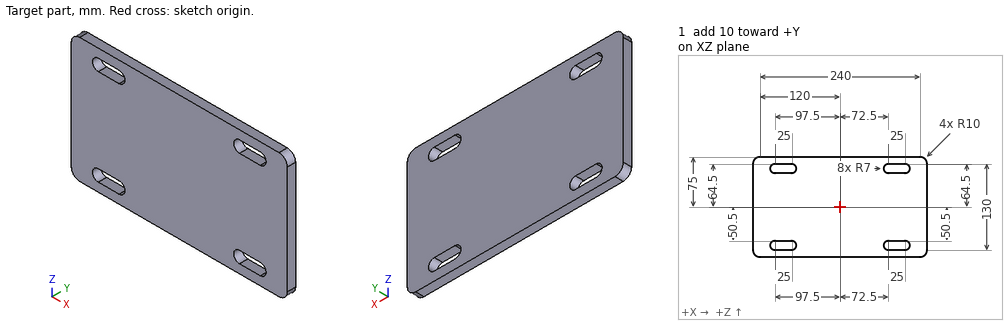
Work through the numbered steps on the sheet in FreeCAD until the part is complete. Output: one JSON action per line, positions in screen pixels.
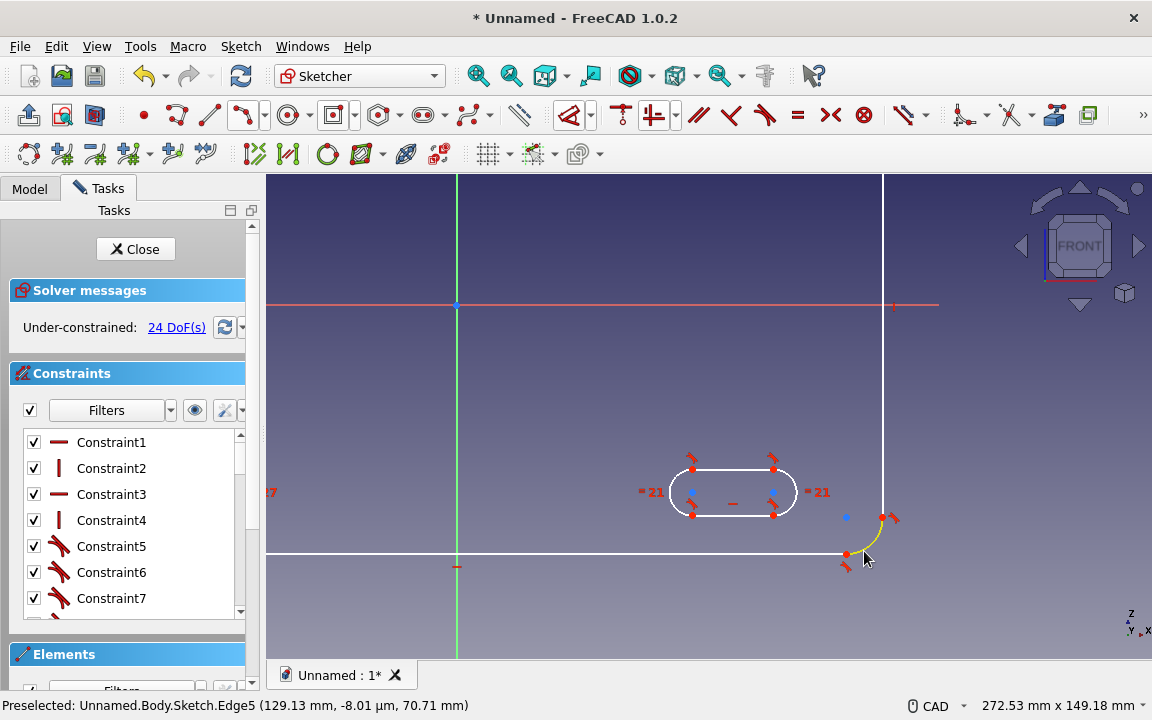
{"action": "left_click", "coordinate": [863, 550]}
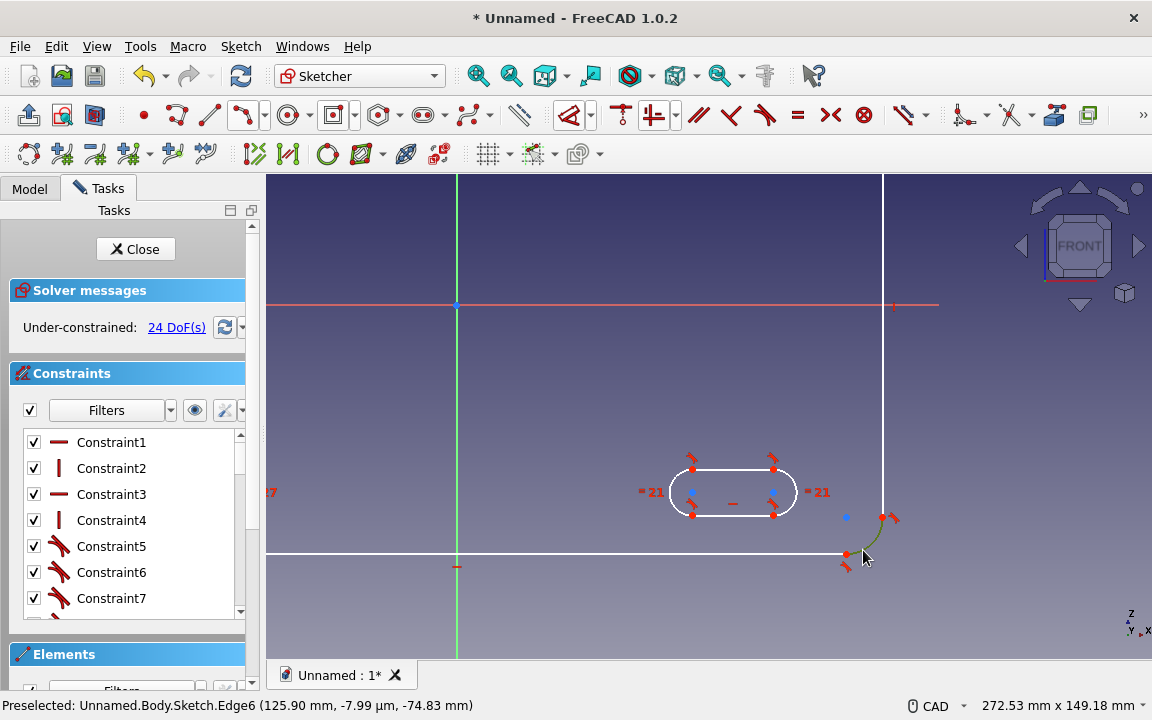
{"action": "scroll", "coordinate": [864, 552], "scroll_direction": "down", "scroll_amount": 3}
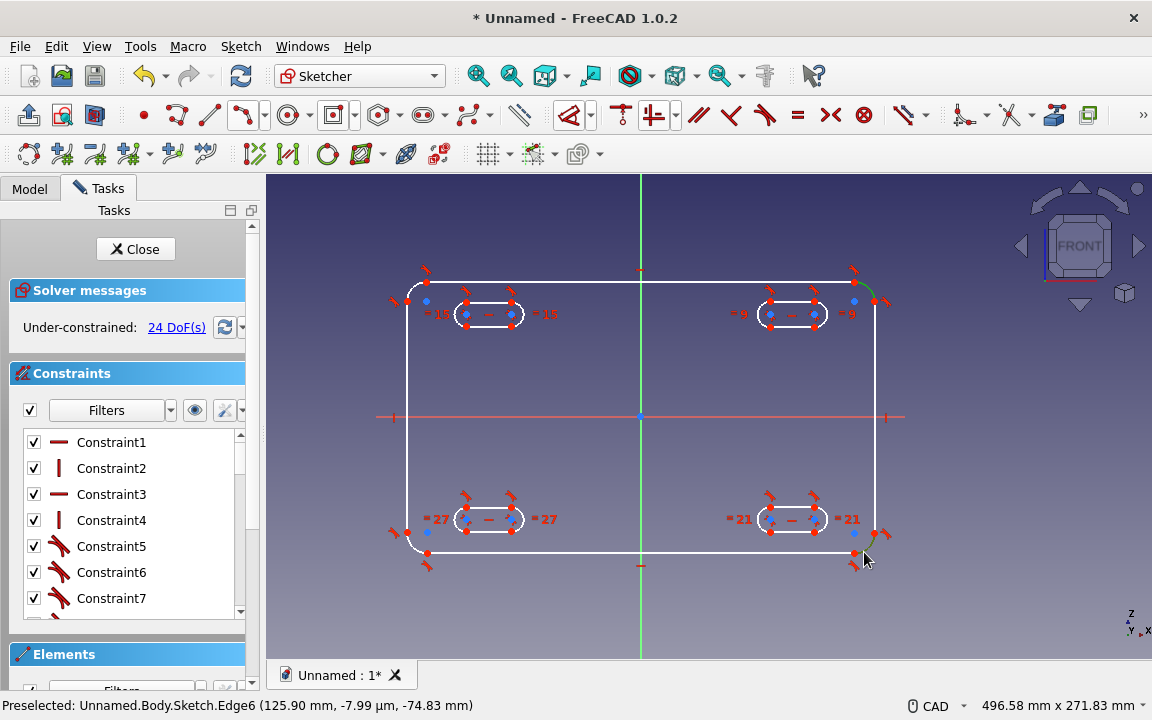
{"action": "scroll", "coordinate": [409, 542], "scroll_direction": "up", "scroll_amount": 2}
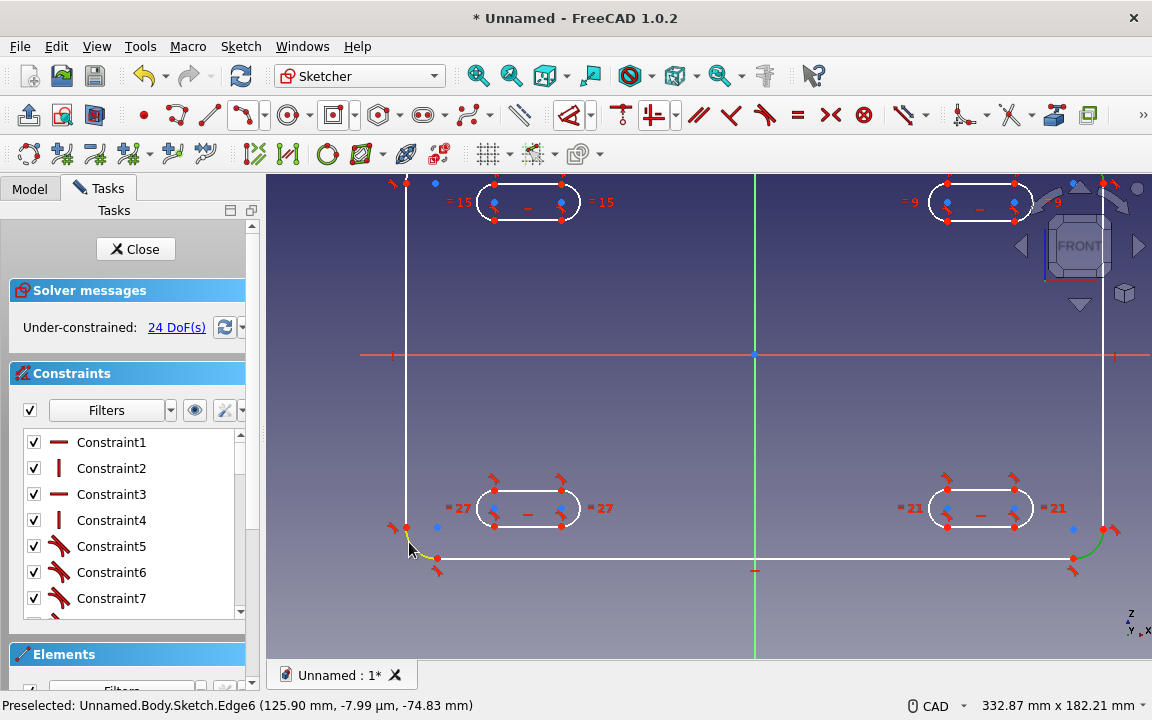
{"action": "left_click", "coordinate": [409, 542]}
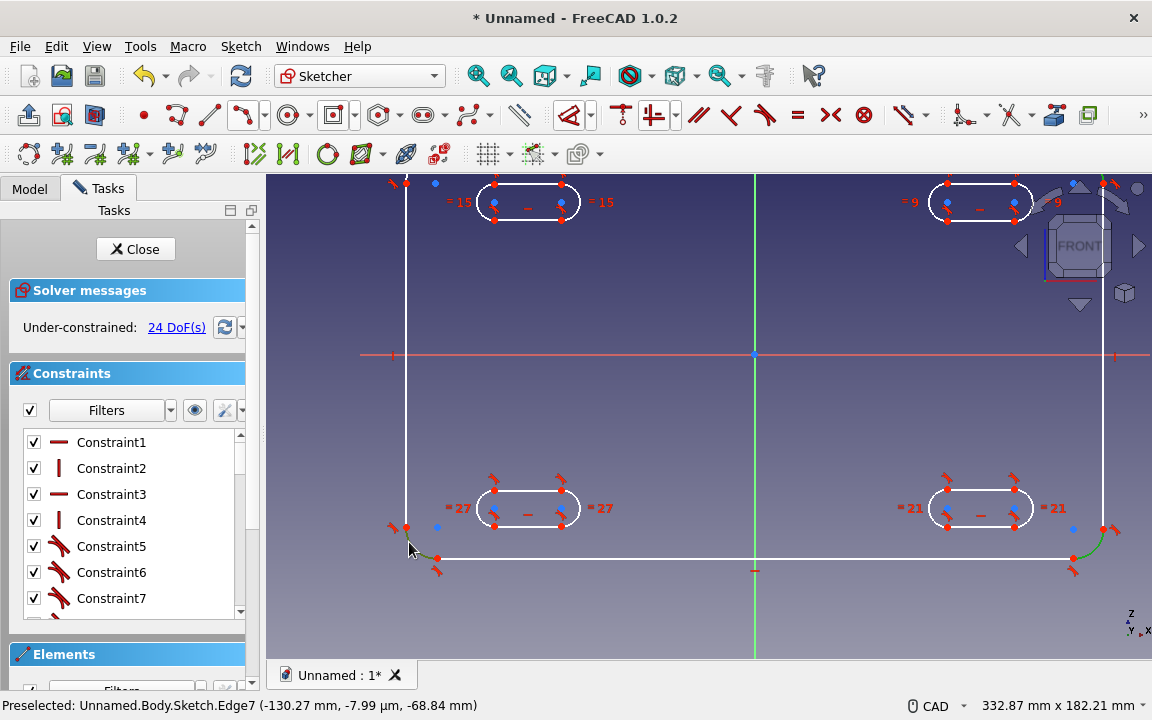
{"action": "scroll", "coordinate": [408, 542], "scroll_direction": "down", "scroll_amount": 2}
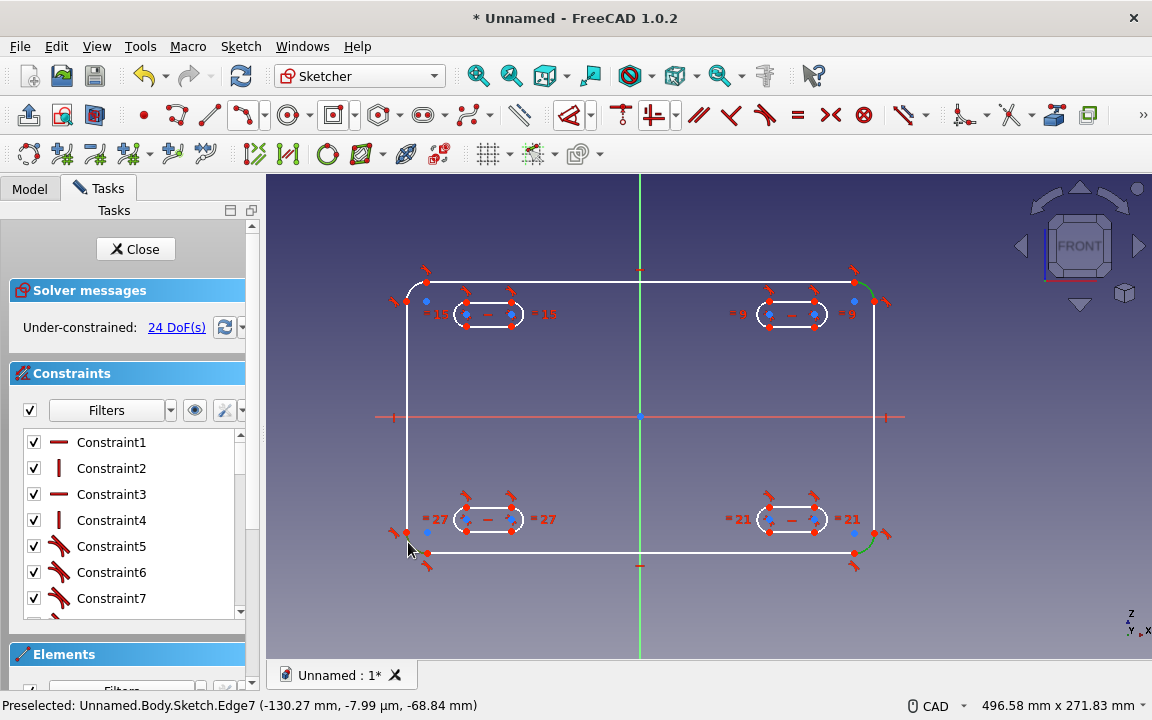
{"action": "scroll", "coordinate": [417, 284], "scroll_direction": "up", "scroll_amount": 3}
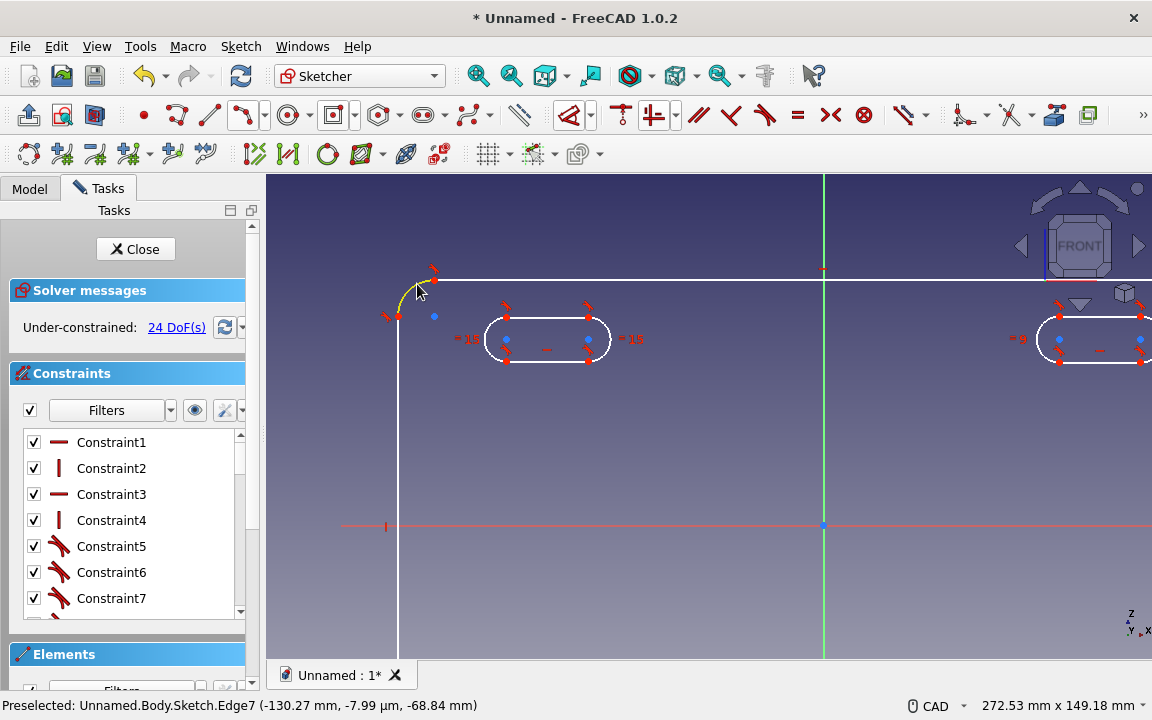
{"action": "left_click", "coordinate": [418, 284]}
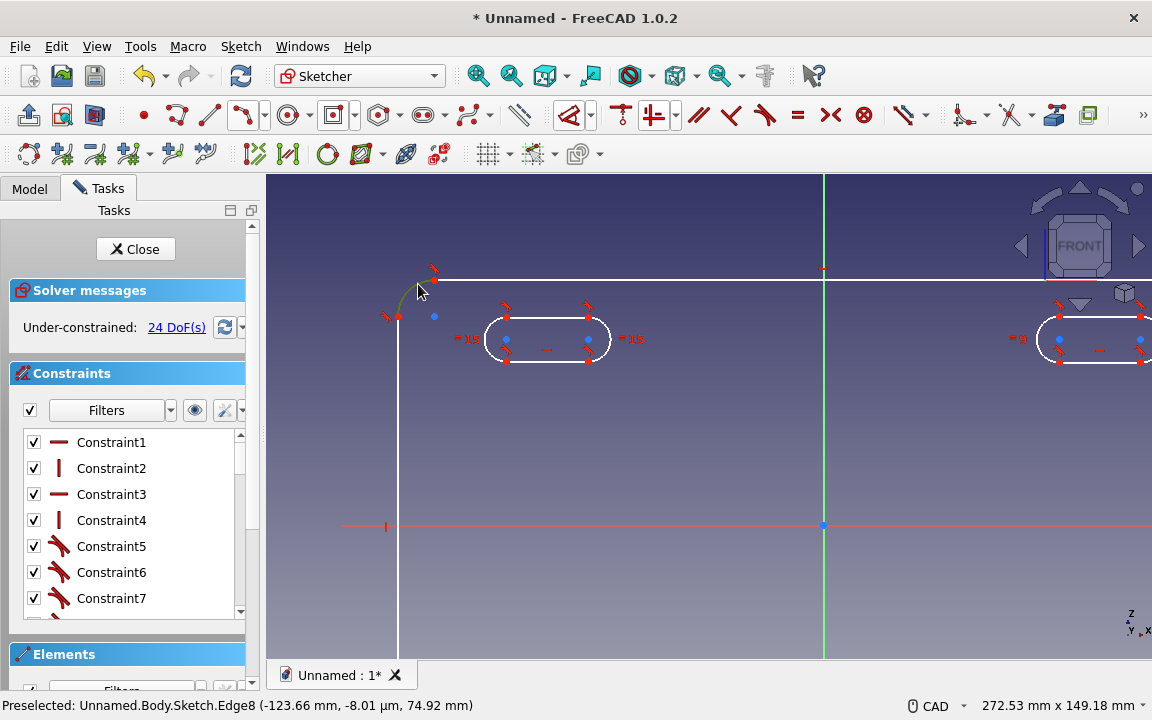
{"action": "left_click", "coordinate": [798, 116]}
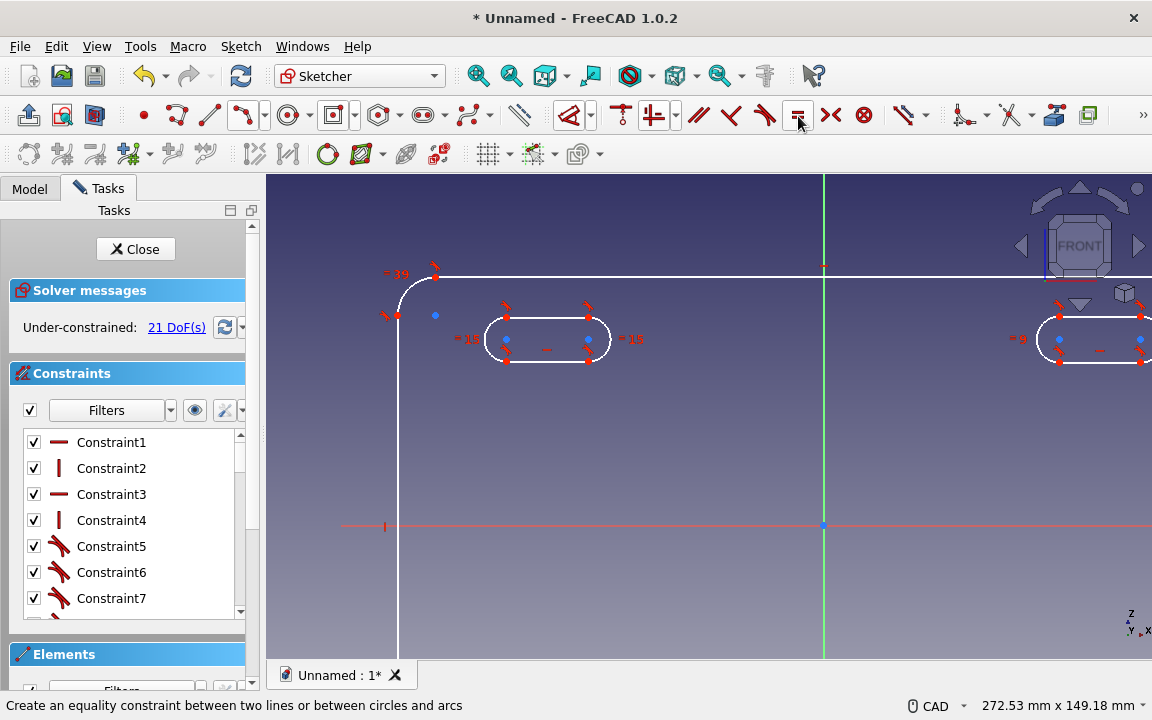
{"action": "scroll", "coordinate": [417, 283], "scroll_direction": "down", "scroll_amount": 3}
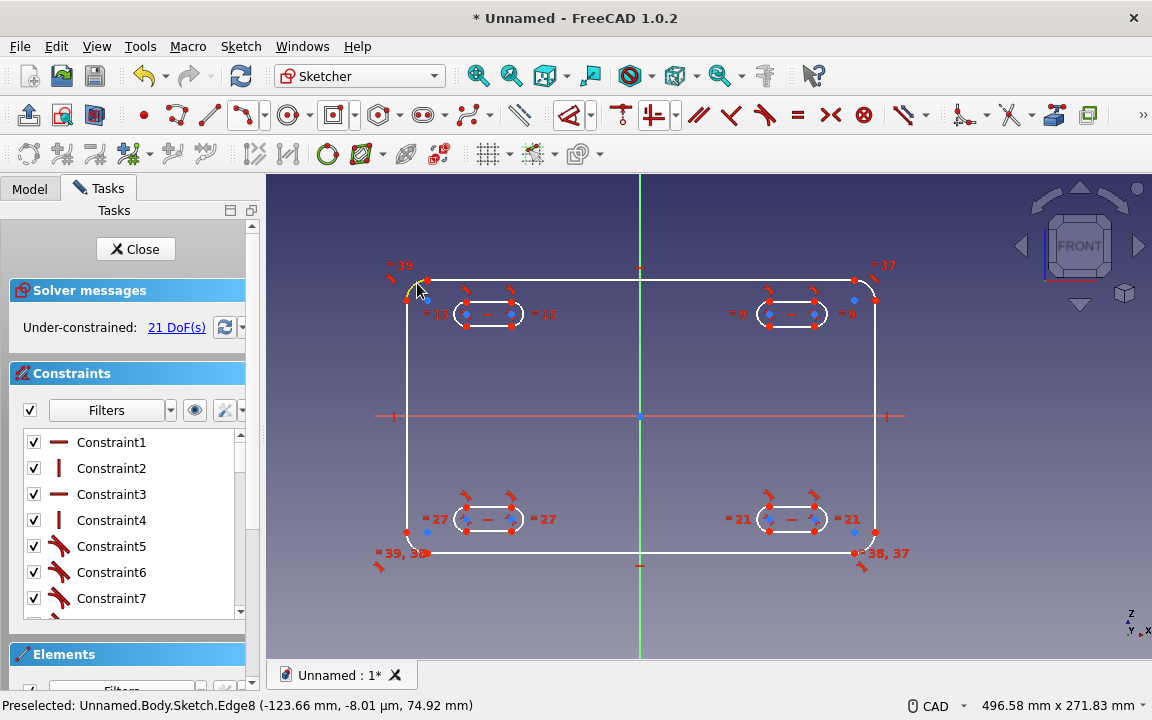
{"action": "left_click", "coordinate": [760, 307]}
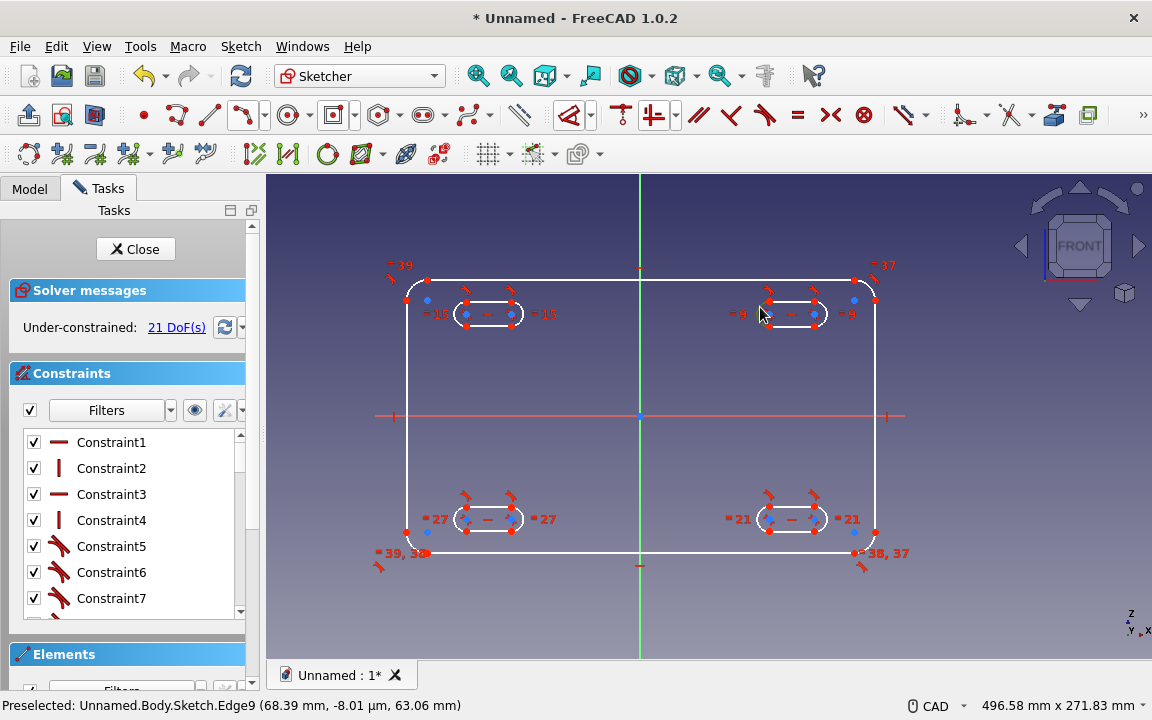
{"action": "scroll", "coordinate": [456, 307], "scroll_direction": "up", "scroll_amount": 2}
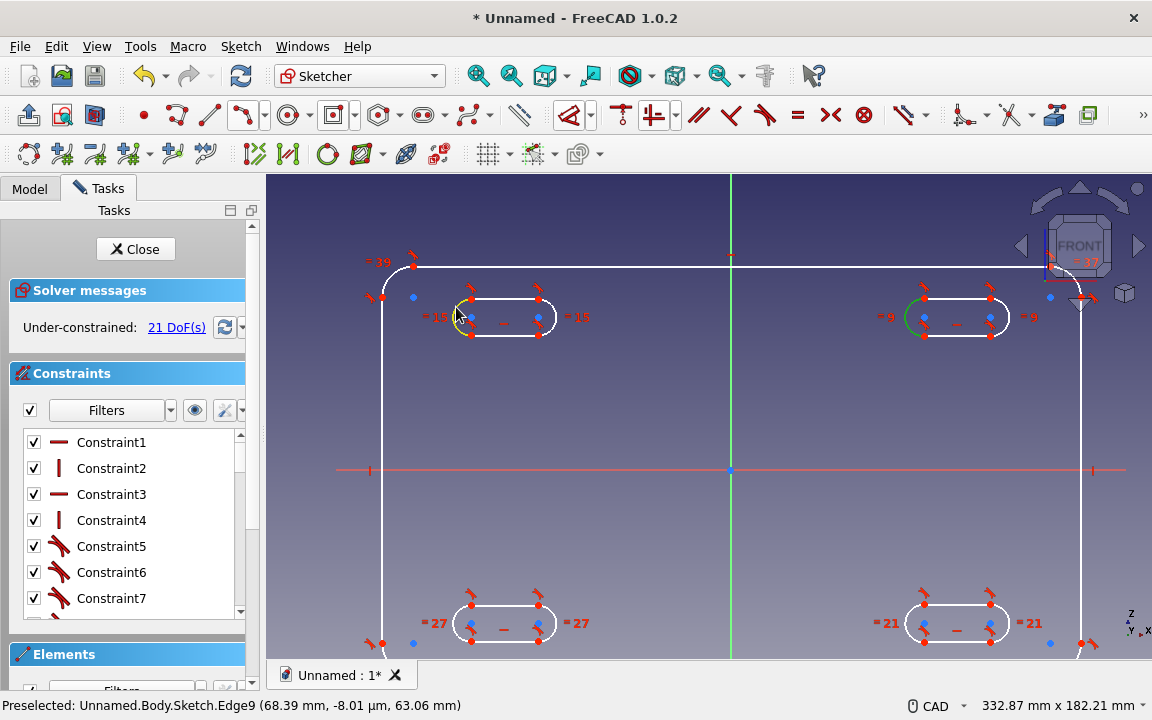
{"action": "left_click", "coordinate": [457, 307]}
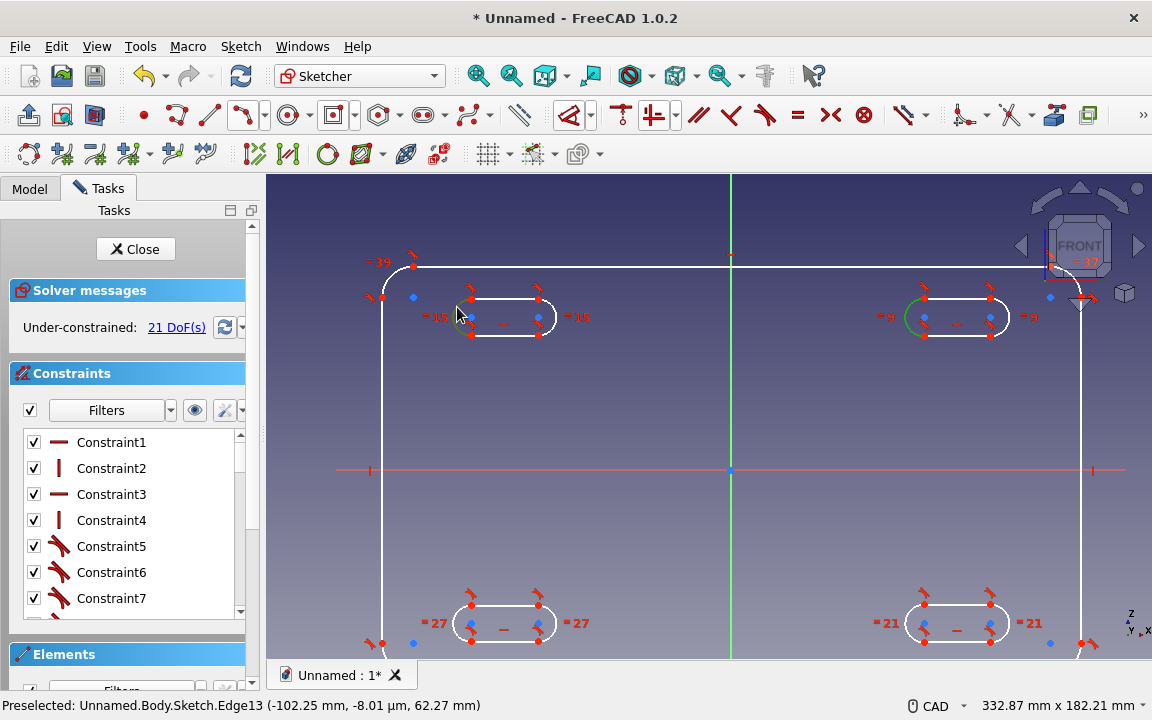
{"action": "left_click", "coordinate": [909, 613]}